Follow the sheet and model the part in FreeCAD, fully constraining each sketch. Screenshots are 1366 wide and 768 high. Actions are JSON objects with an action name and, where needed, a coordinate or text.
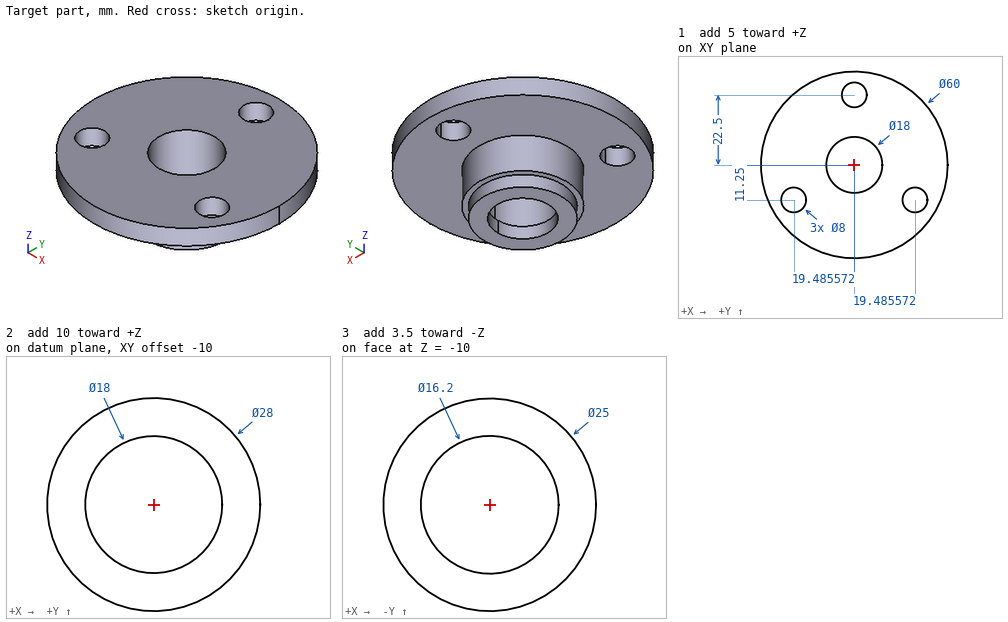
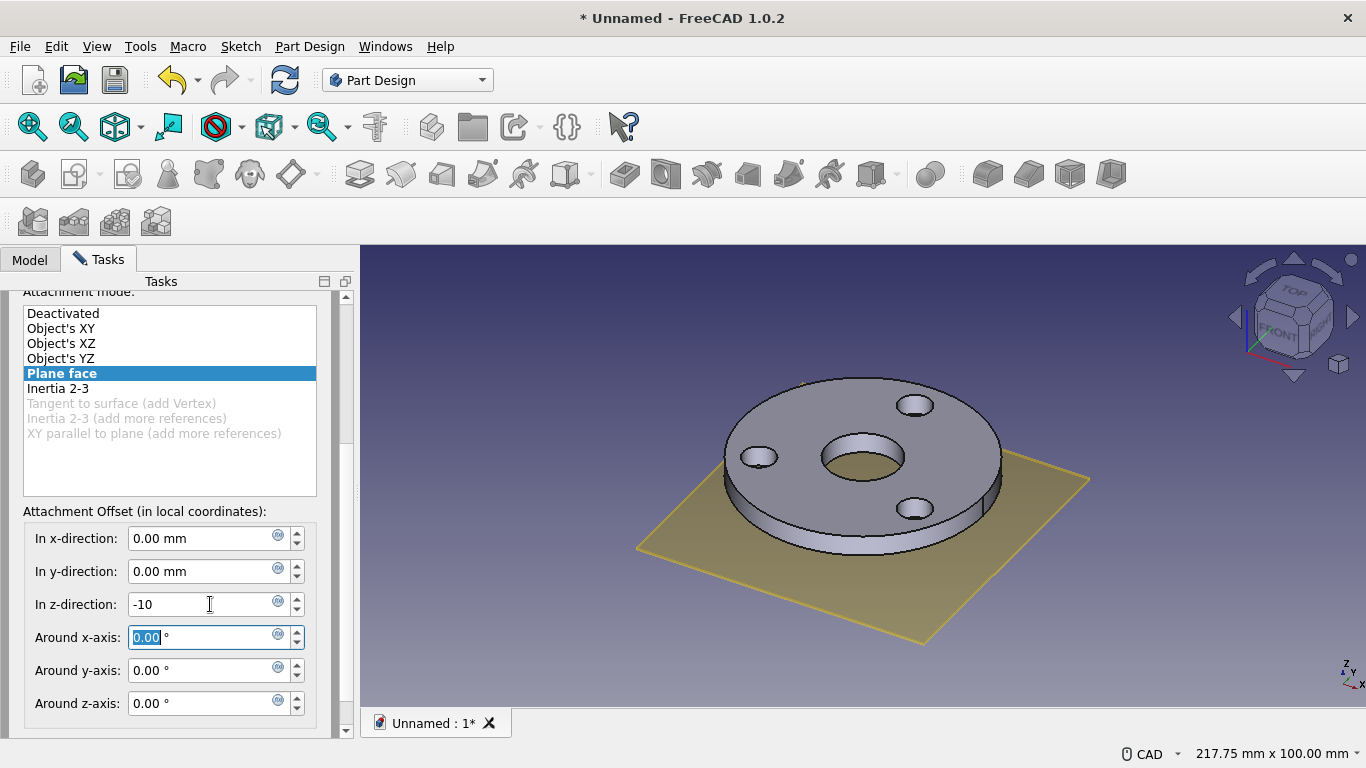
{"action": "scroll", "coordinate": [346, 514], "scroll_direction": "up", "scroll_amount": 5}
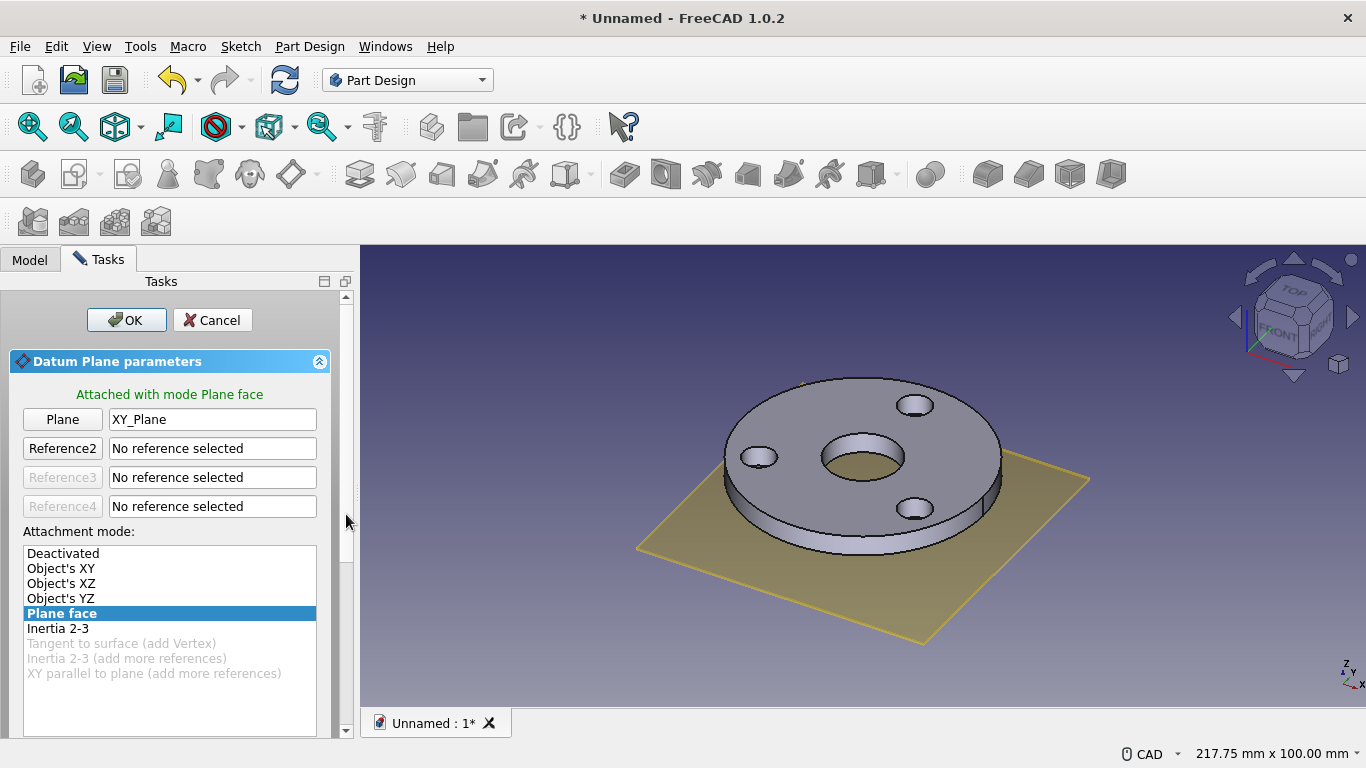
{"action": "left_click", "coordinate": [127, 320]}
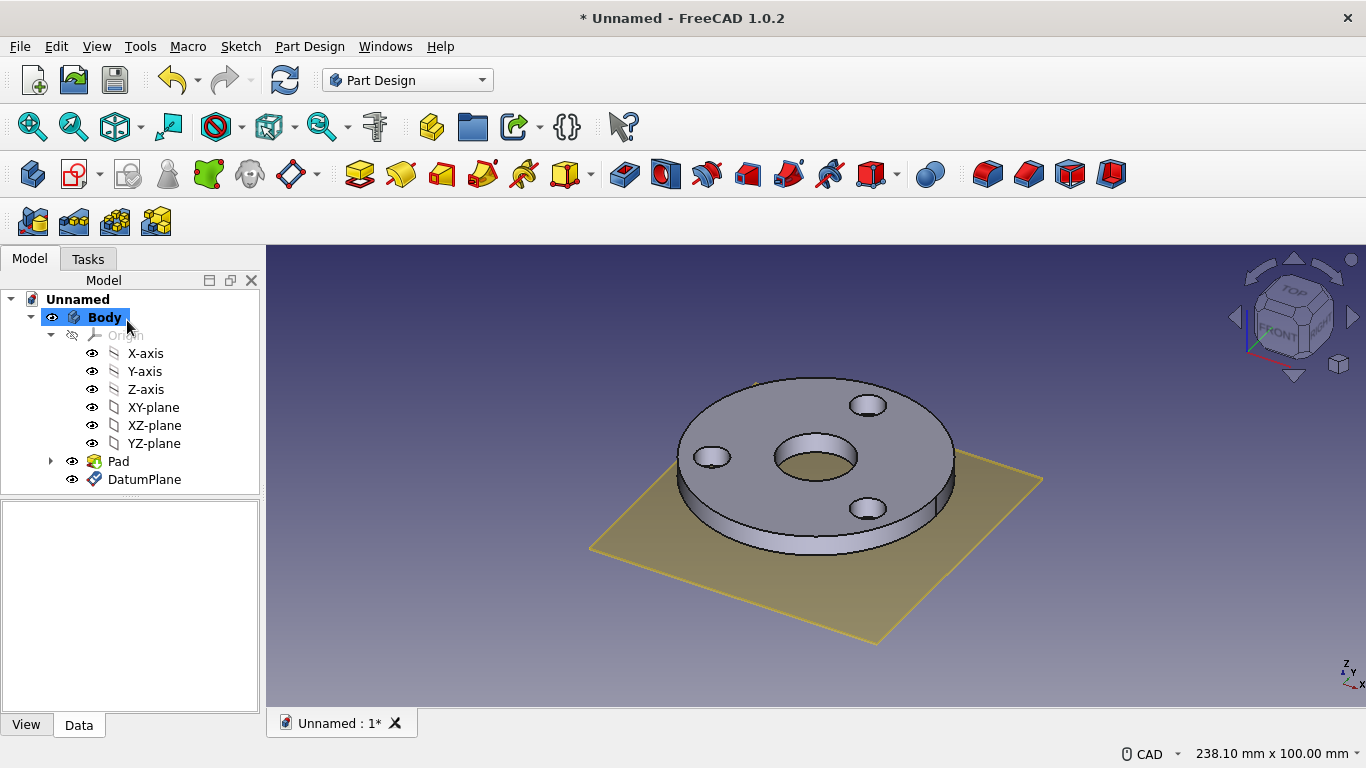
{"action": "left_click", "coordinate": [117, 479]}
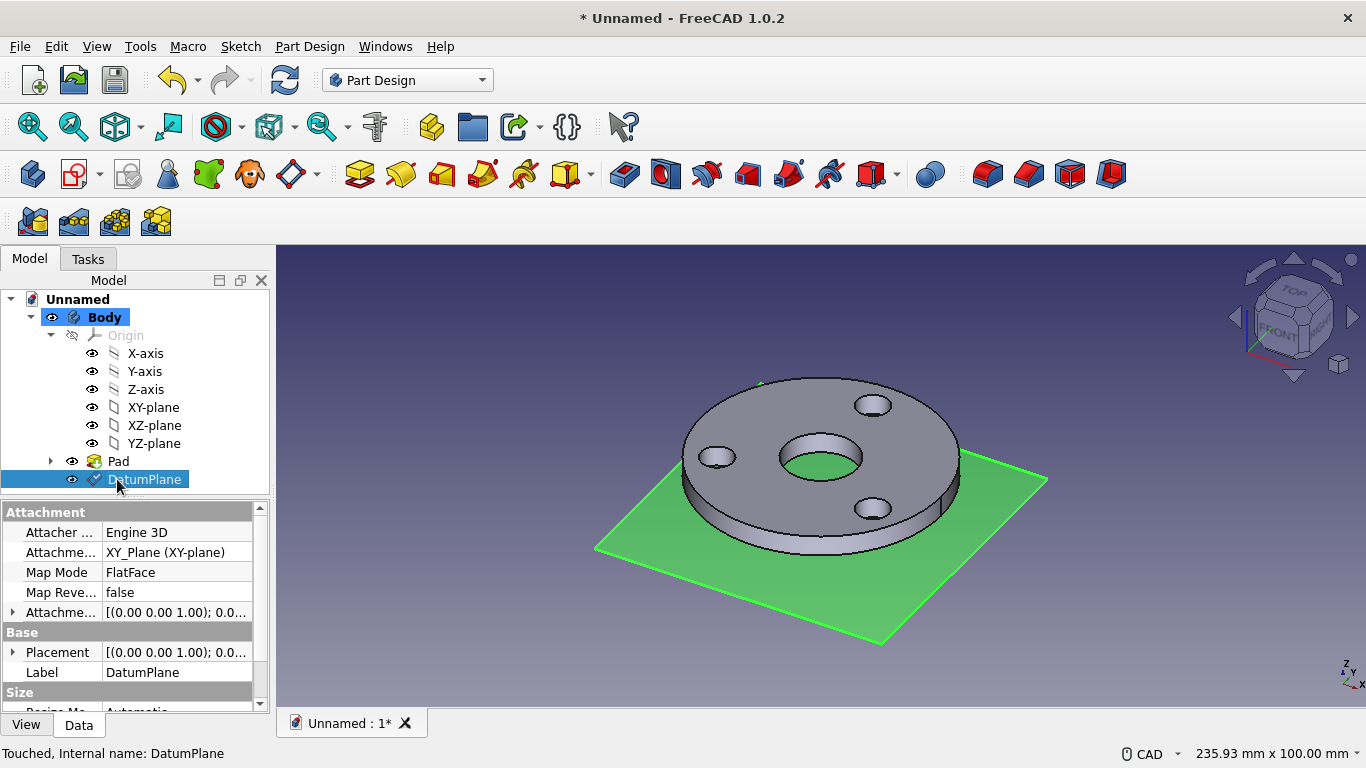
{"action": "left_click", "coordinate": [74, 174]}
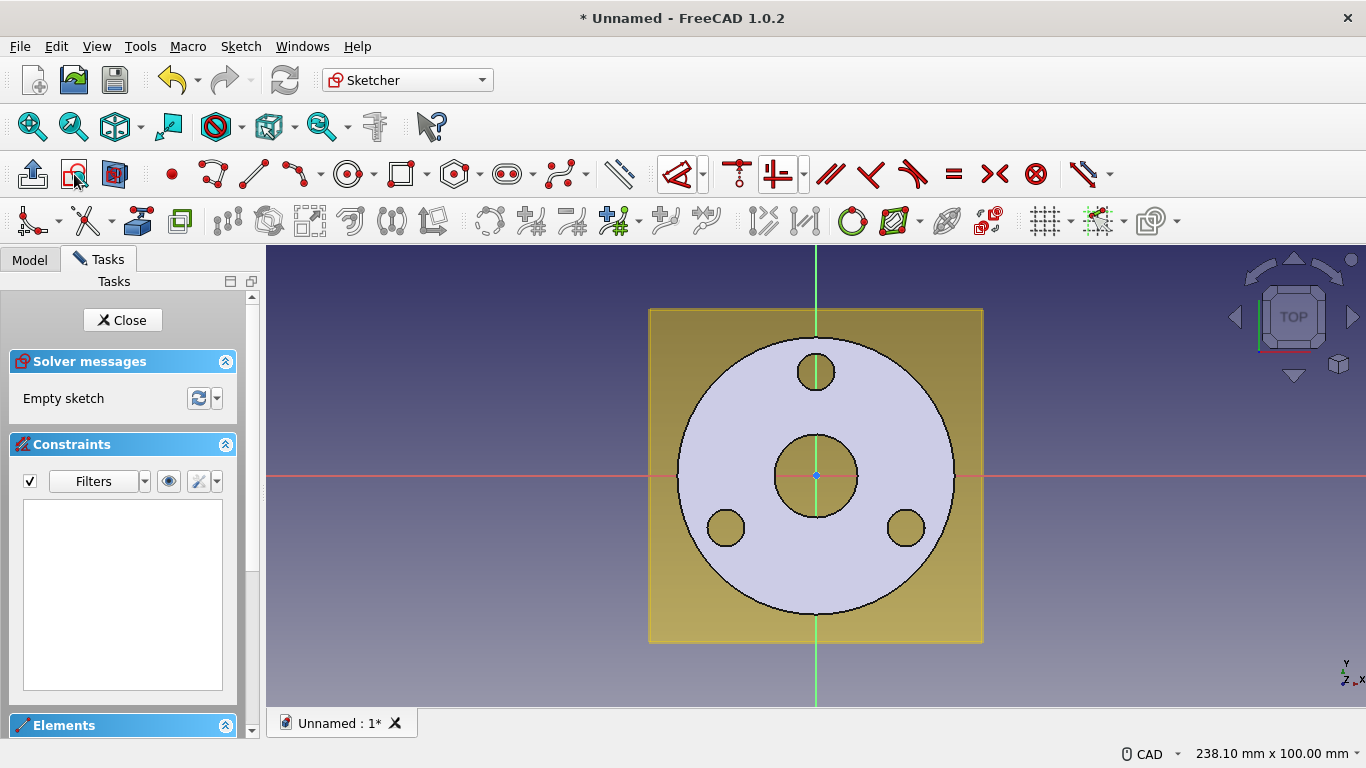
{"action": "key", "text": "q s"}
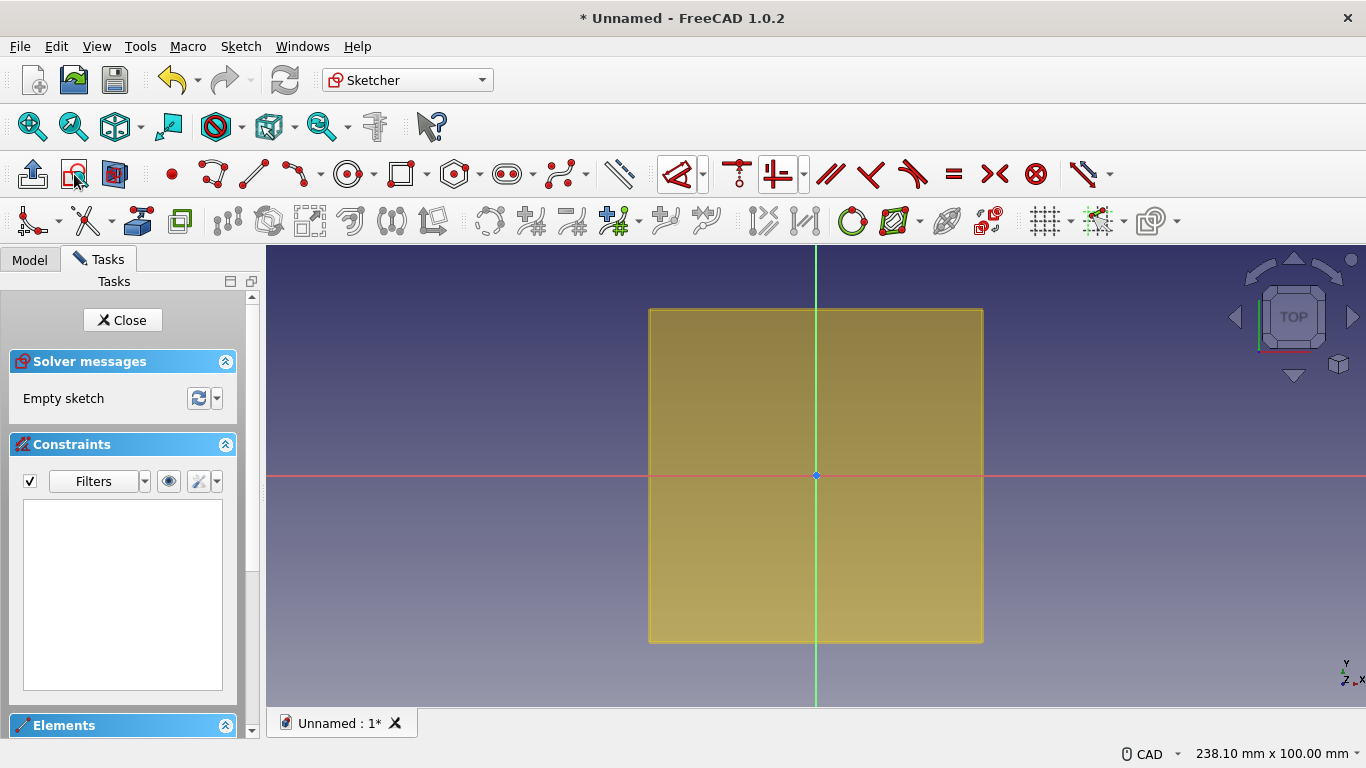
{"action": "scroll", "coordinate": [872, 476], "scroll_direction": "up", "scroll_amount": 4}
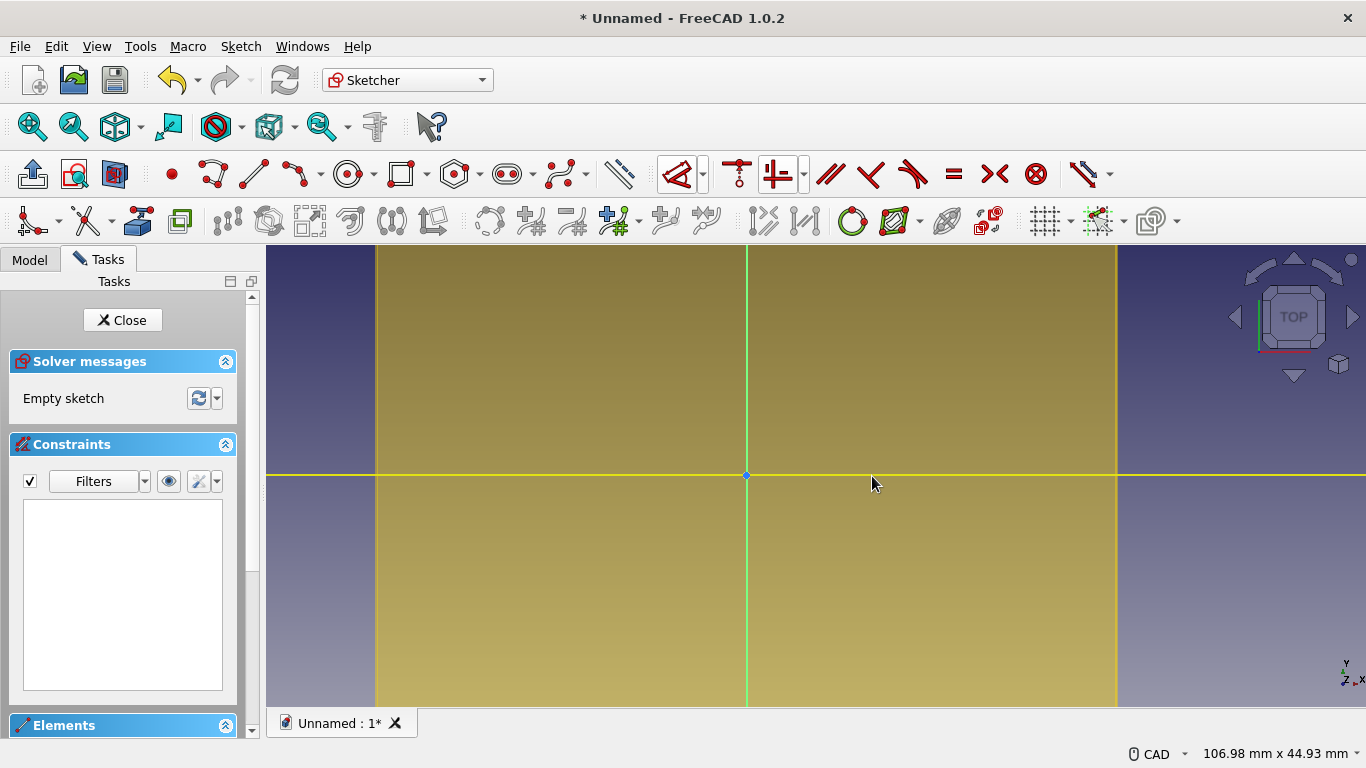
{"action": "left_click", "coordinate": [348, 174]}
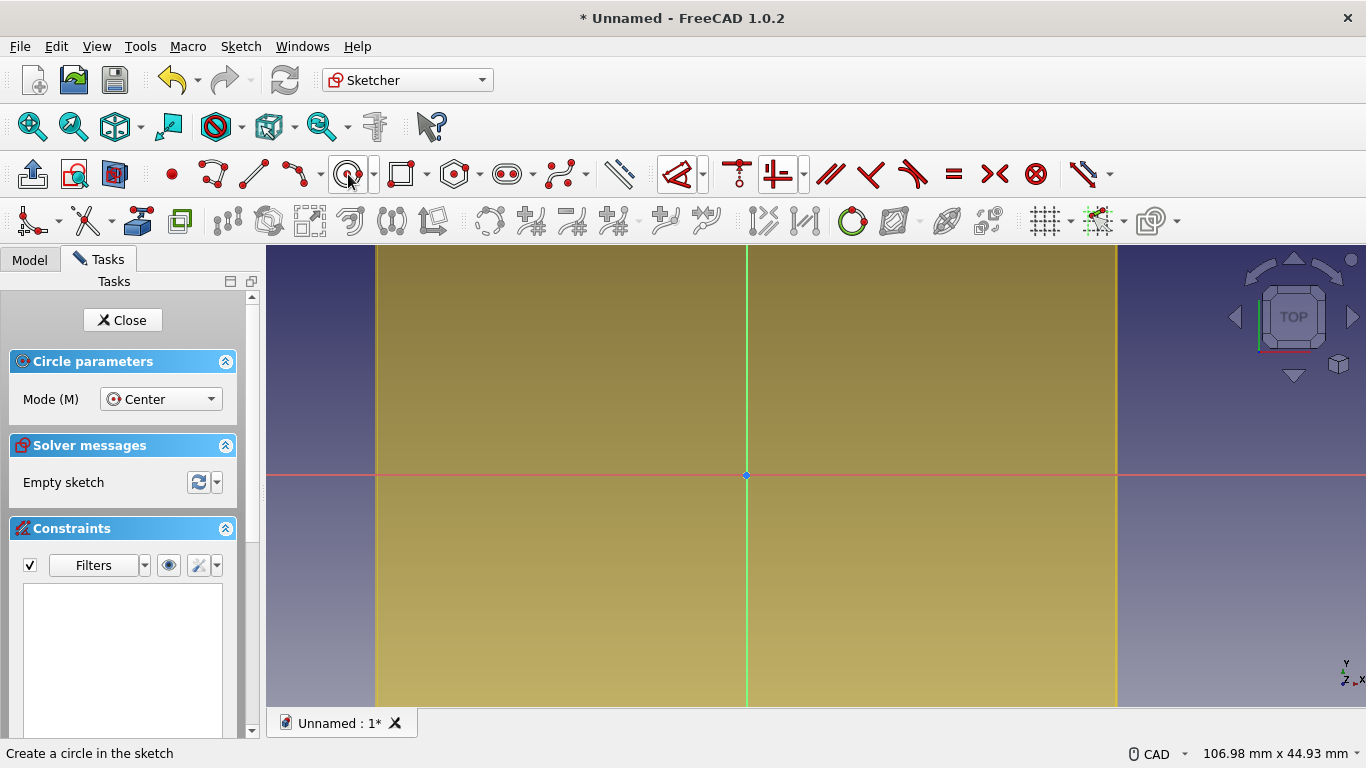
{"action": "left_click", "coordinate": [747, 475]}
{"action": "mouse_move", "coordinate": [848, 374]}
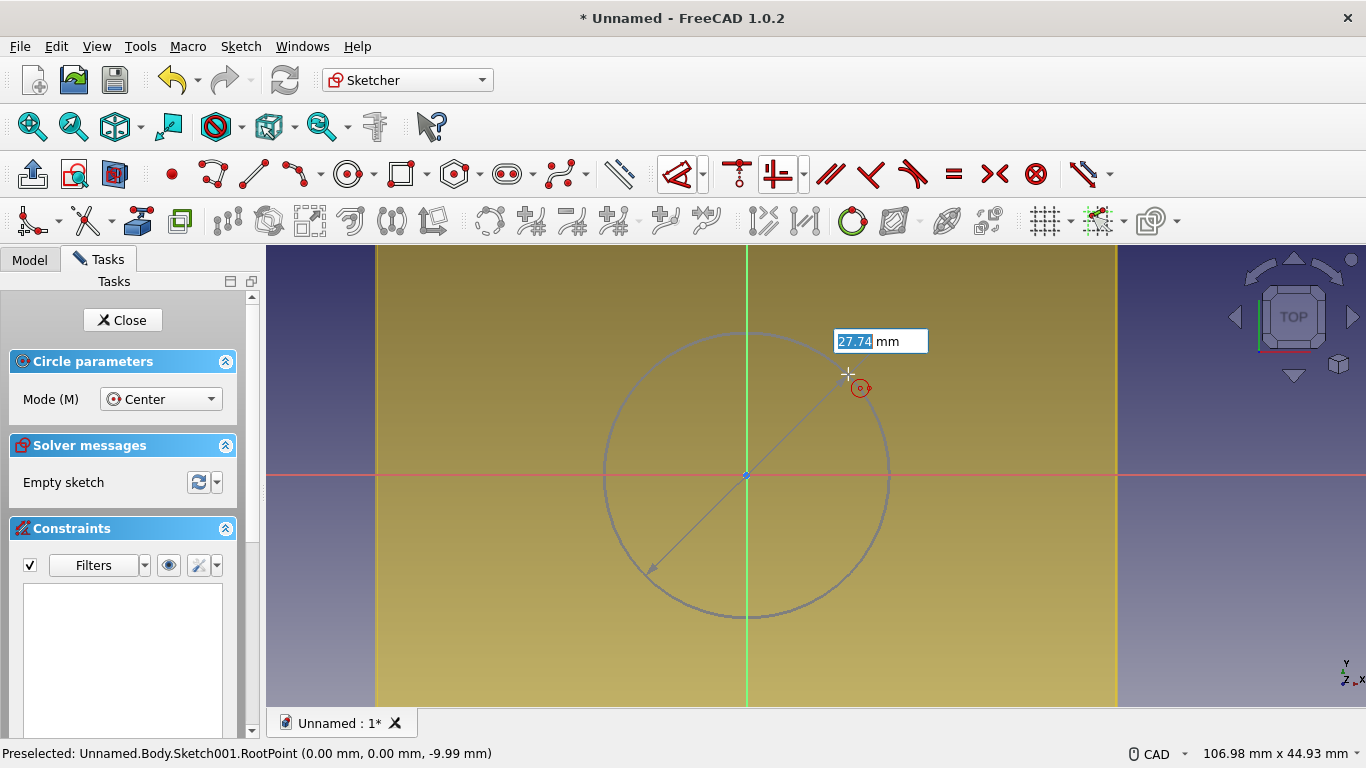
{"action": "type", "text": "28"}
{"action": "key", "text": "Return"}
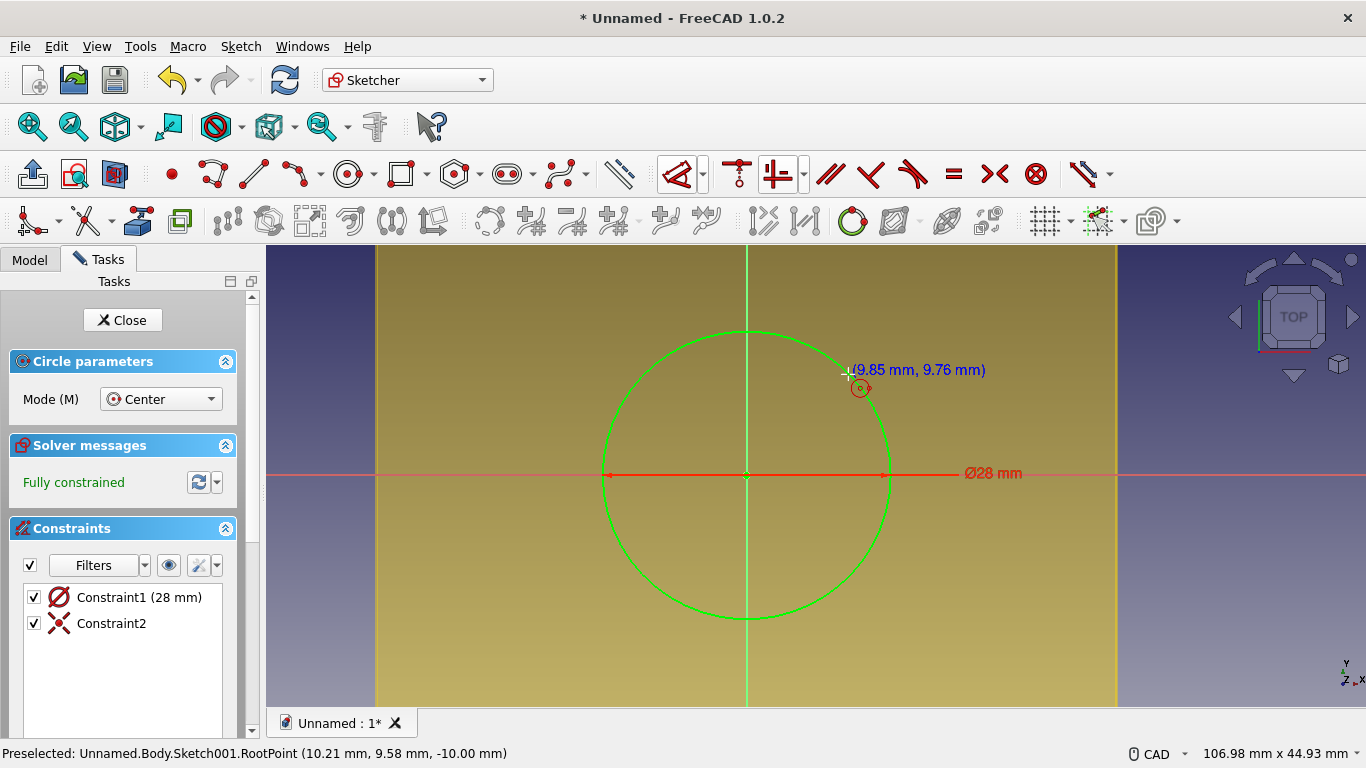
{"action": "left_click", "coordinate": [747, 475]}
{"action": "mouse_move", "coordinate": [812, 410]}